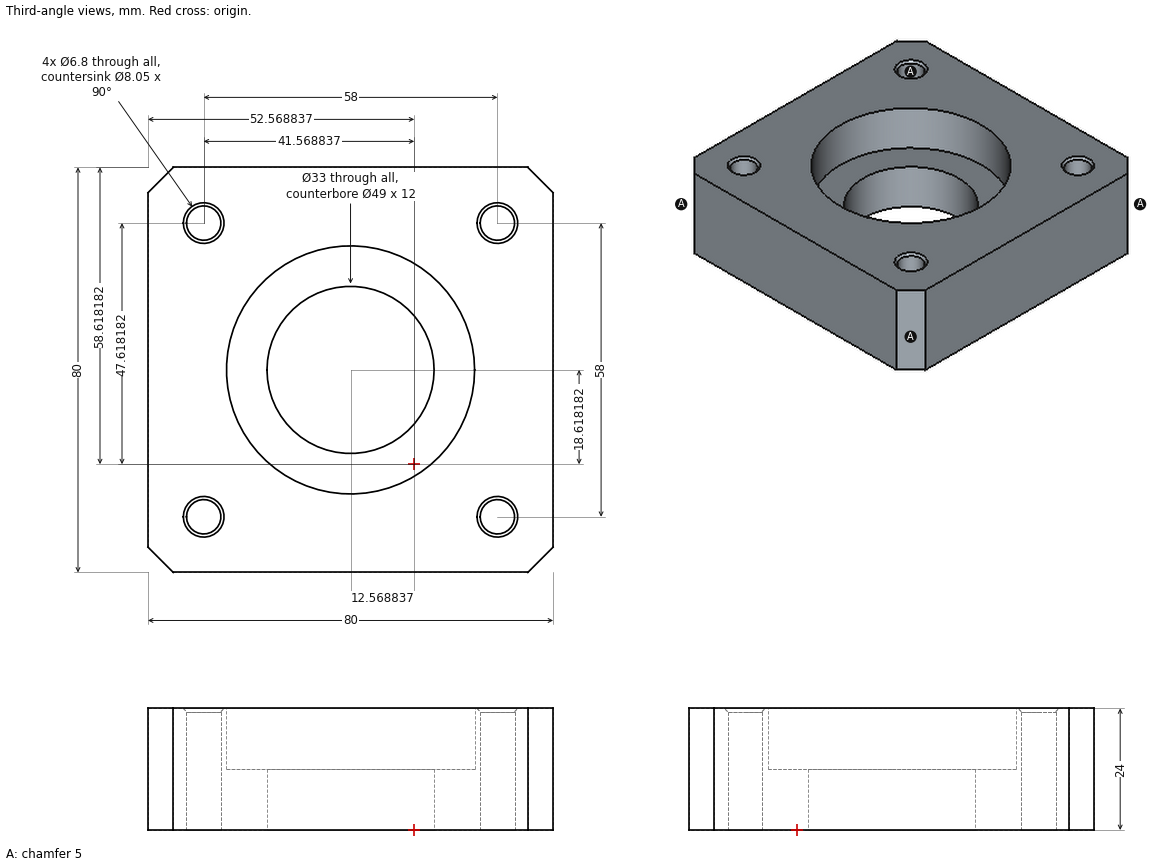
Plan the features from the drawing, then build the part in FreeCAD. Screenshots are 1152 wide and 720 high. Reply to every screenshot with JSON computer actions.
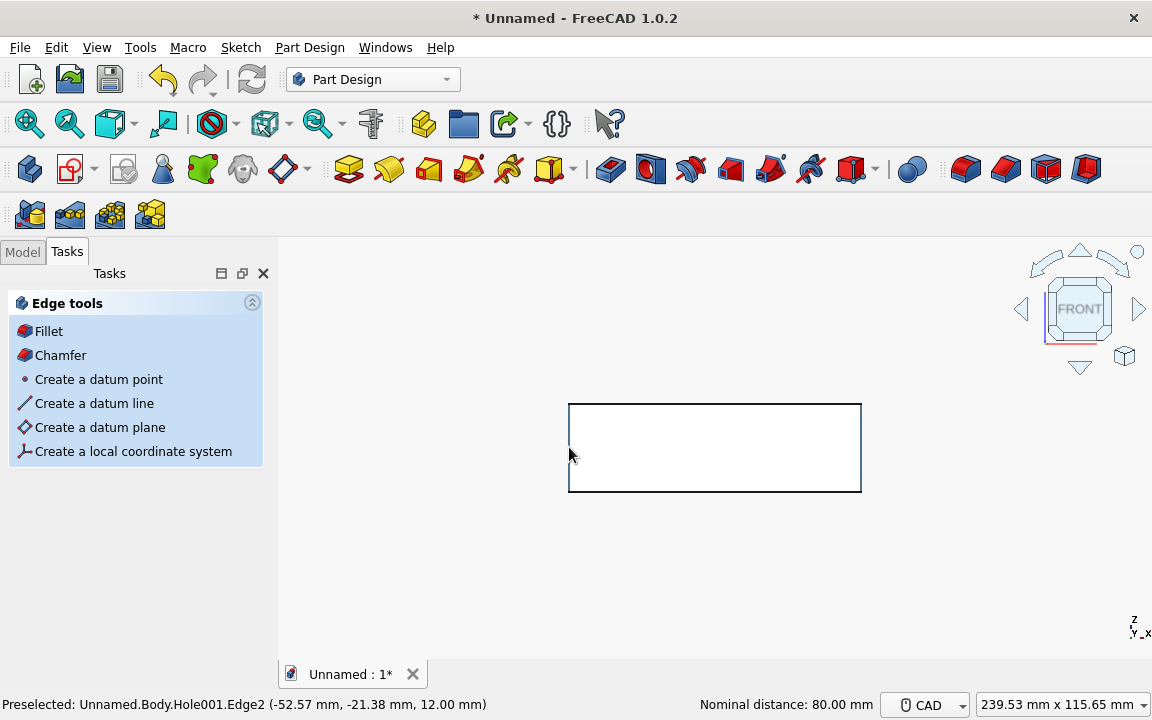
{"action": "key", "text": "3"}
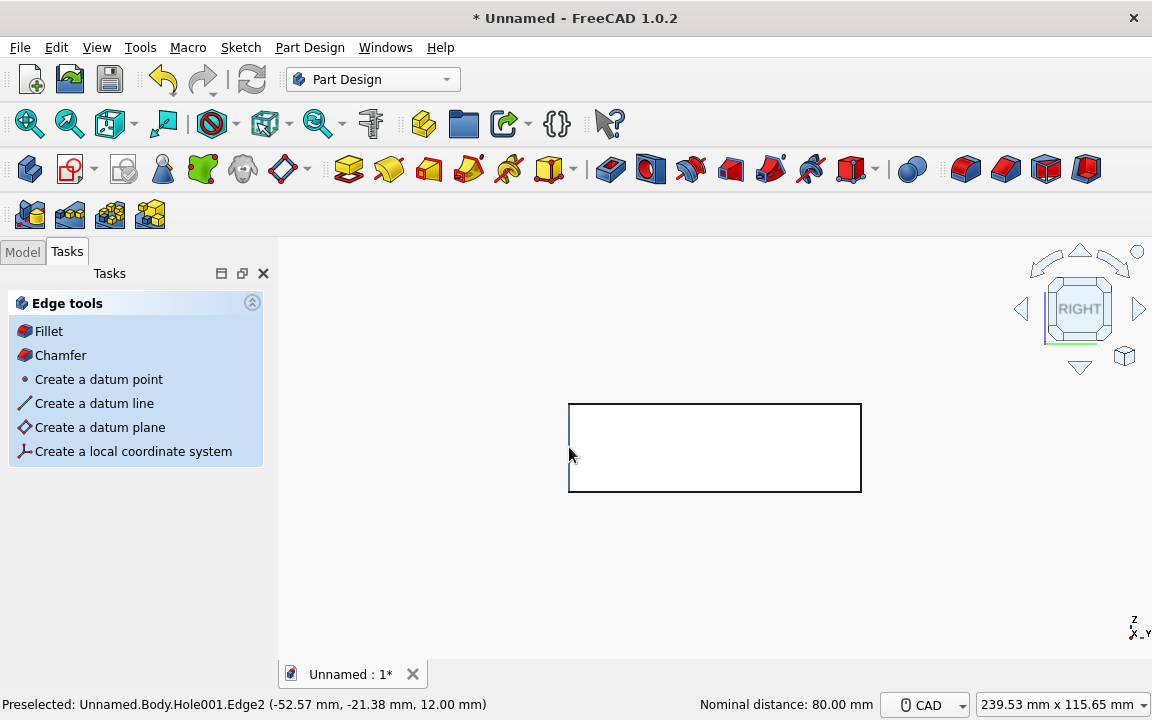
{"action": "left_click", "coordinate": [30, 124]}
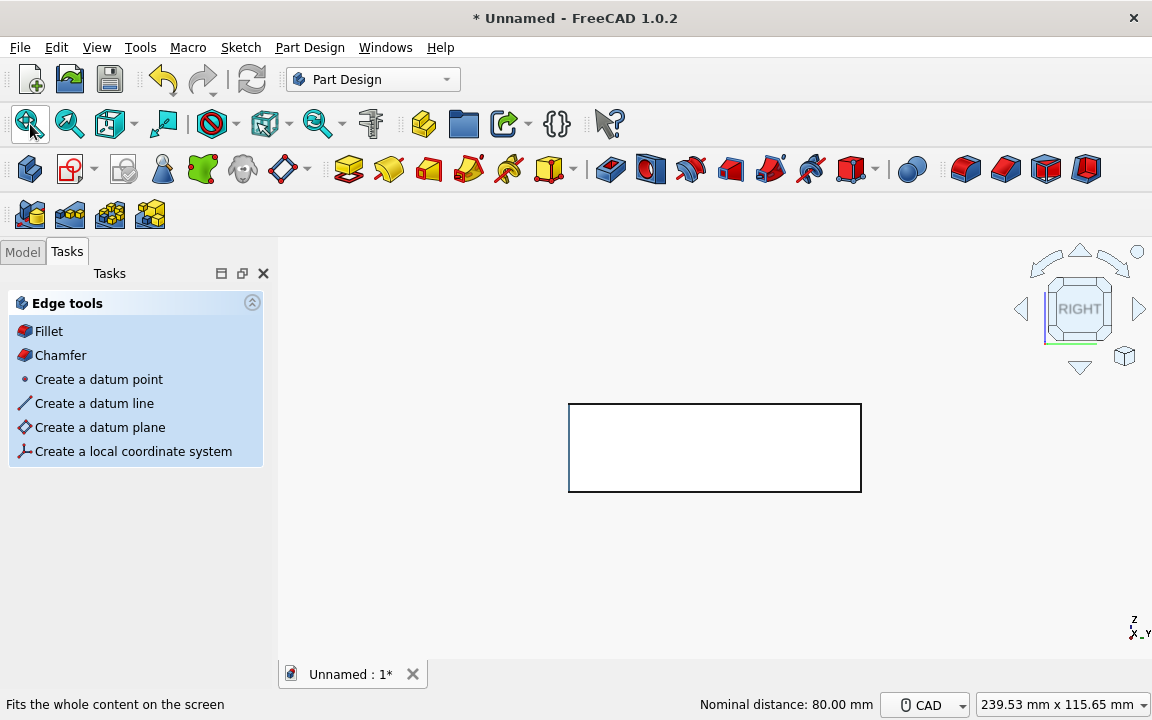
{"action": "left_click", "coordinate": [861, 447], "text": "ctrl"}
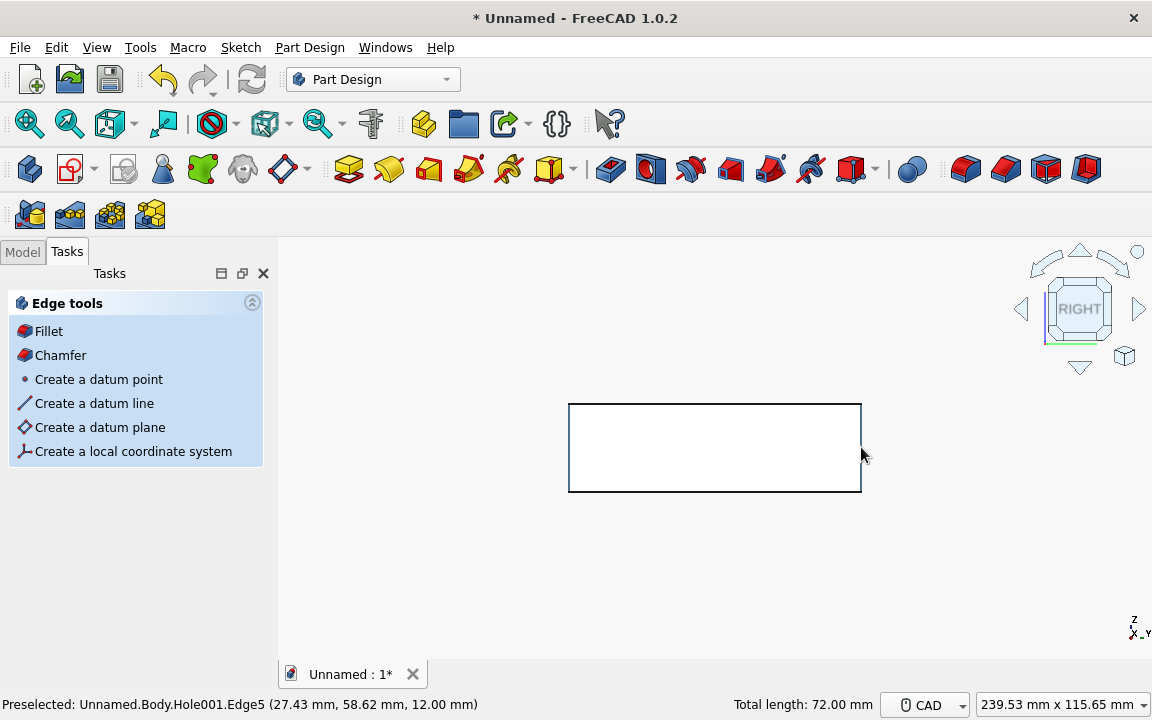
{"action": "key", "text": "5"}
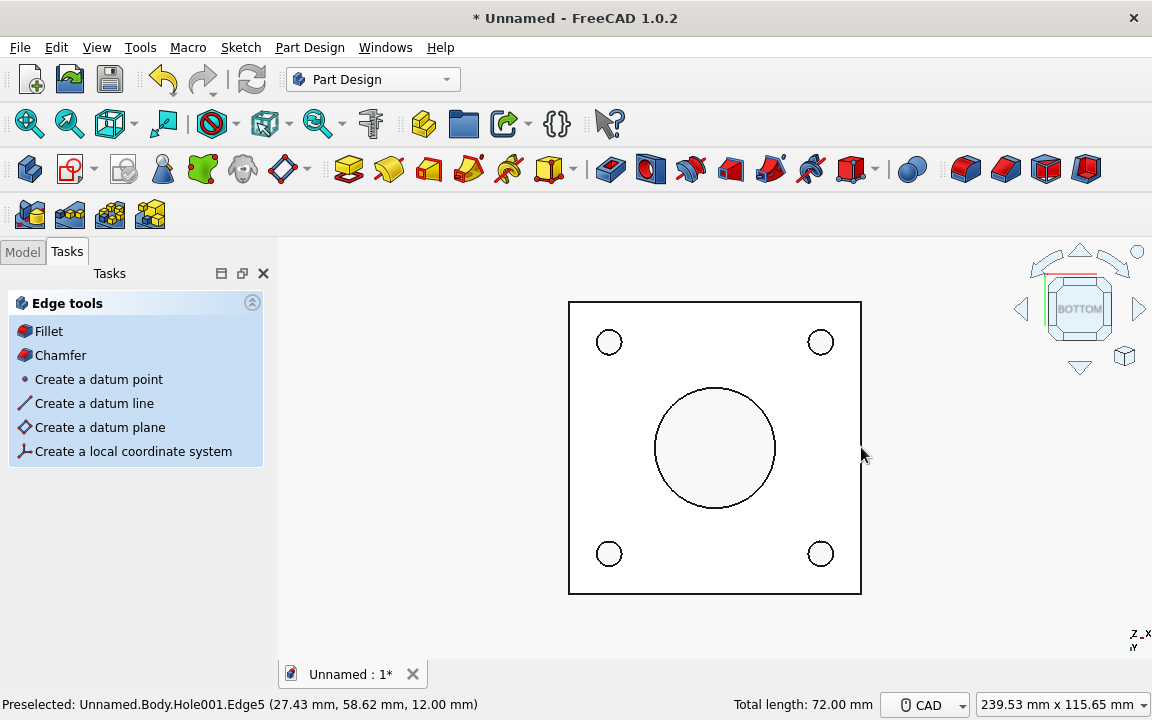
{"action": "key", "text": "4"}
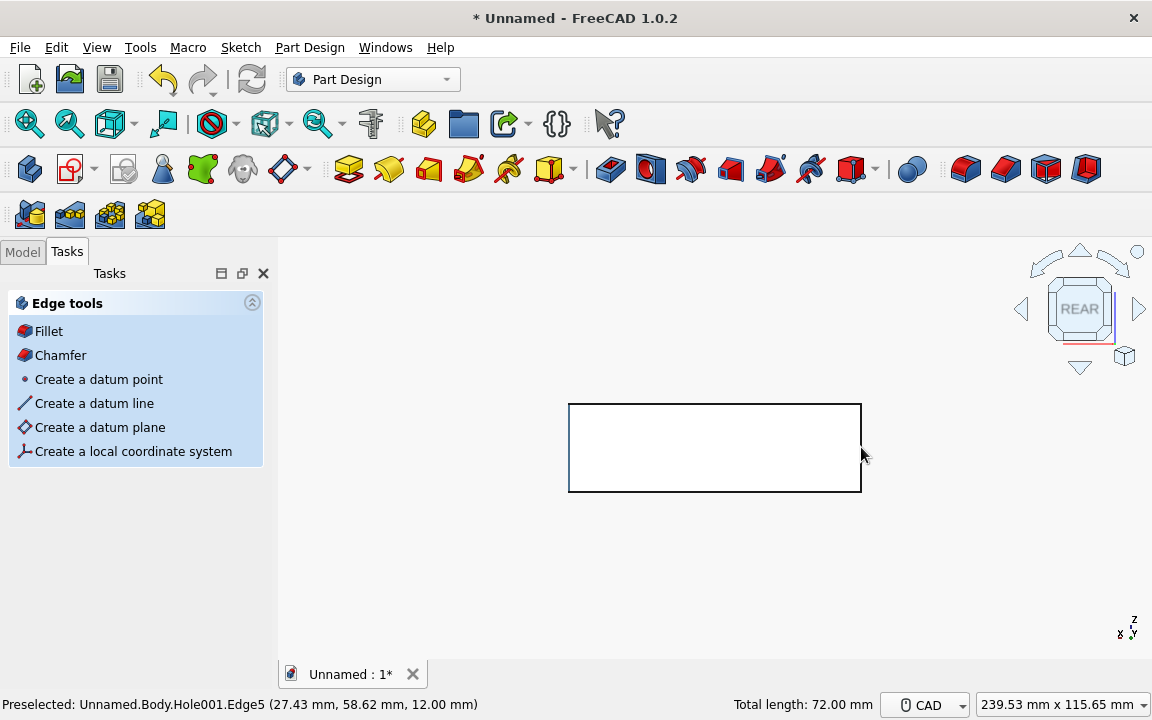
{"action": "left_click", "coordinate": [30, 124]}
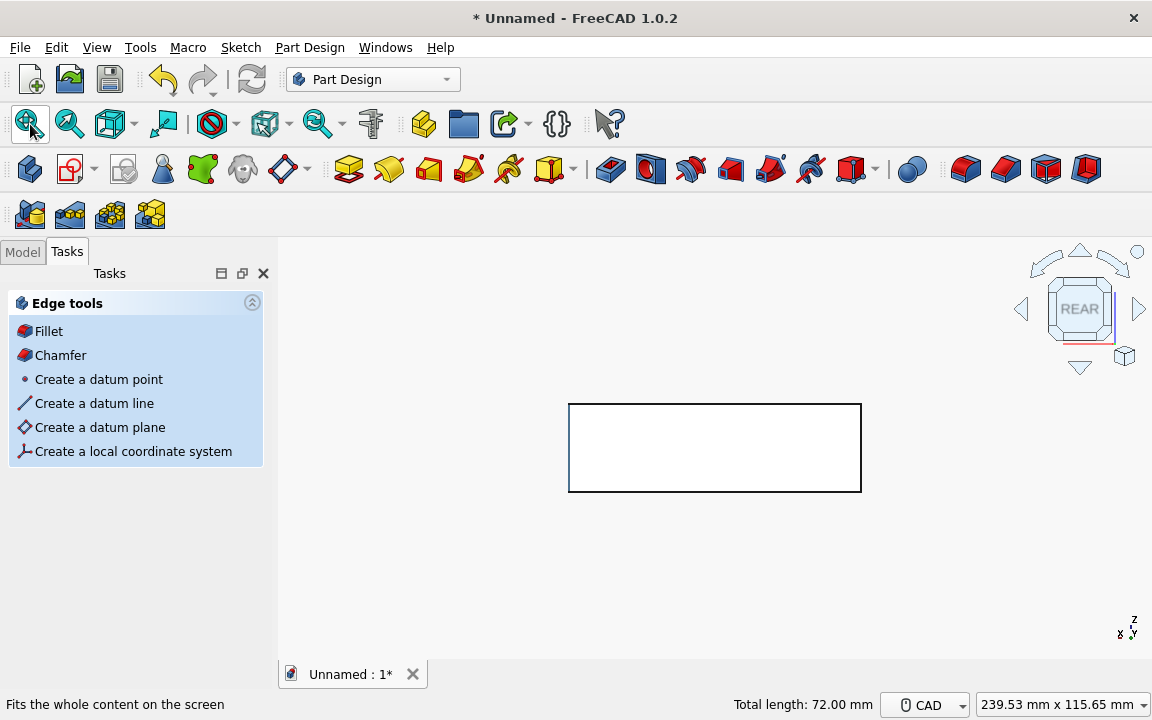
{"action": "left_click", "coordinate": [861, 447], "text": "ctrl"}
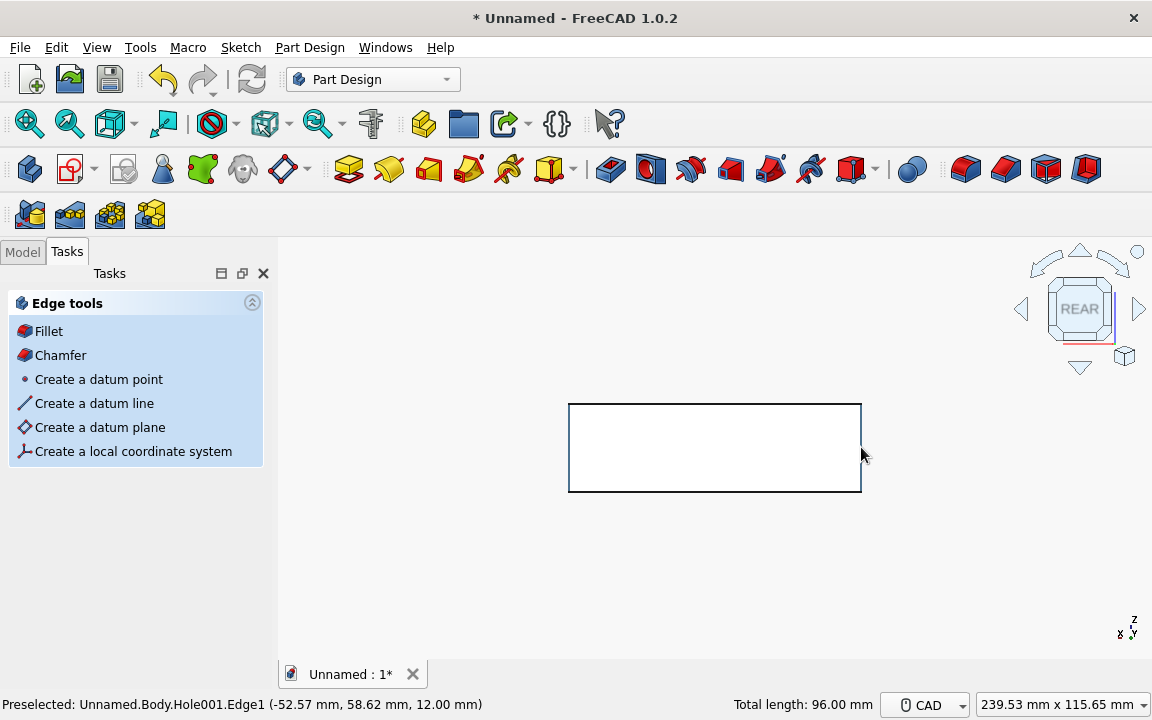
{"action": "left_click", "coordinate": [1006, 170]}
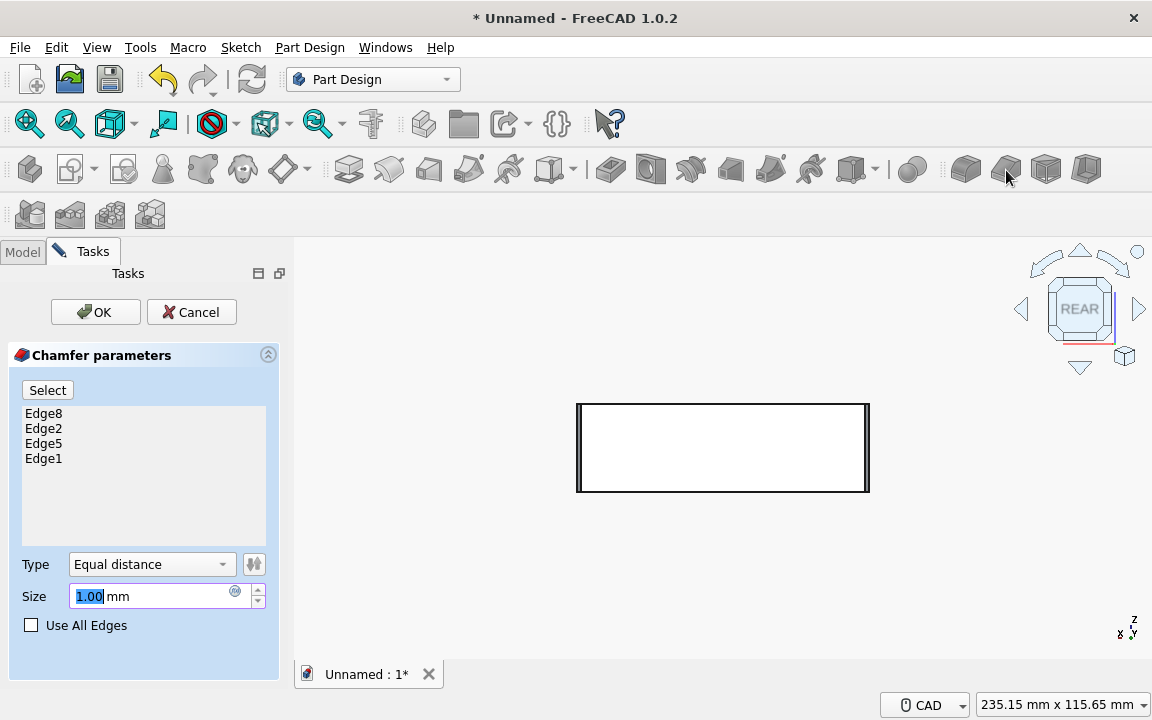
{"action": "type", "text": "5"}
{"action": "key", "text": "Tab"}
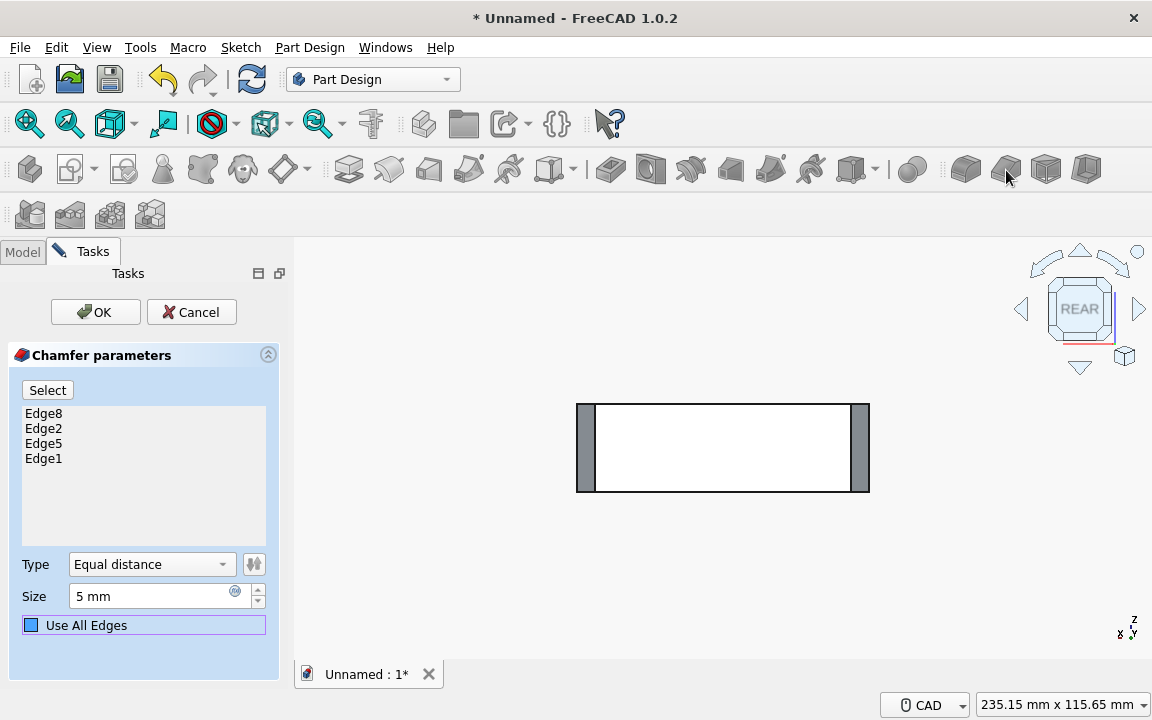
{"action": "left_click", "coordinate": [96, 312]}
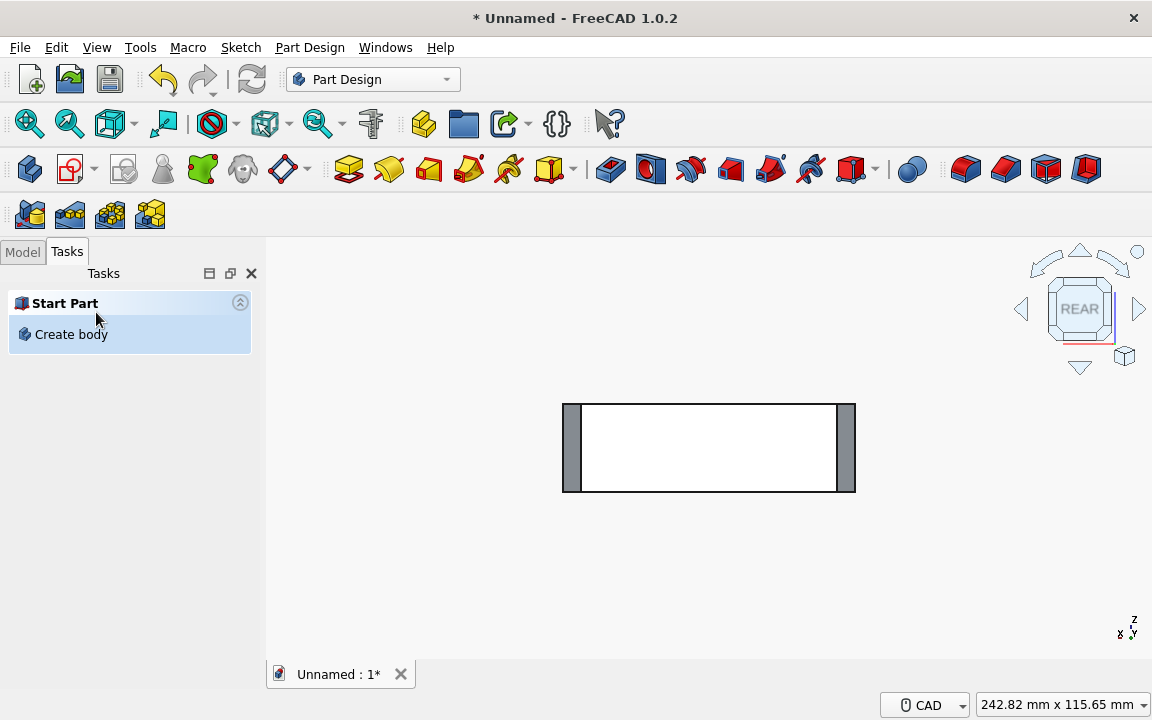
{"action": "key", "text": "0"}